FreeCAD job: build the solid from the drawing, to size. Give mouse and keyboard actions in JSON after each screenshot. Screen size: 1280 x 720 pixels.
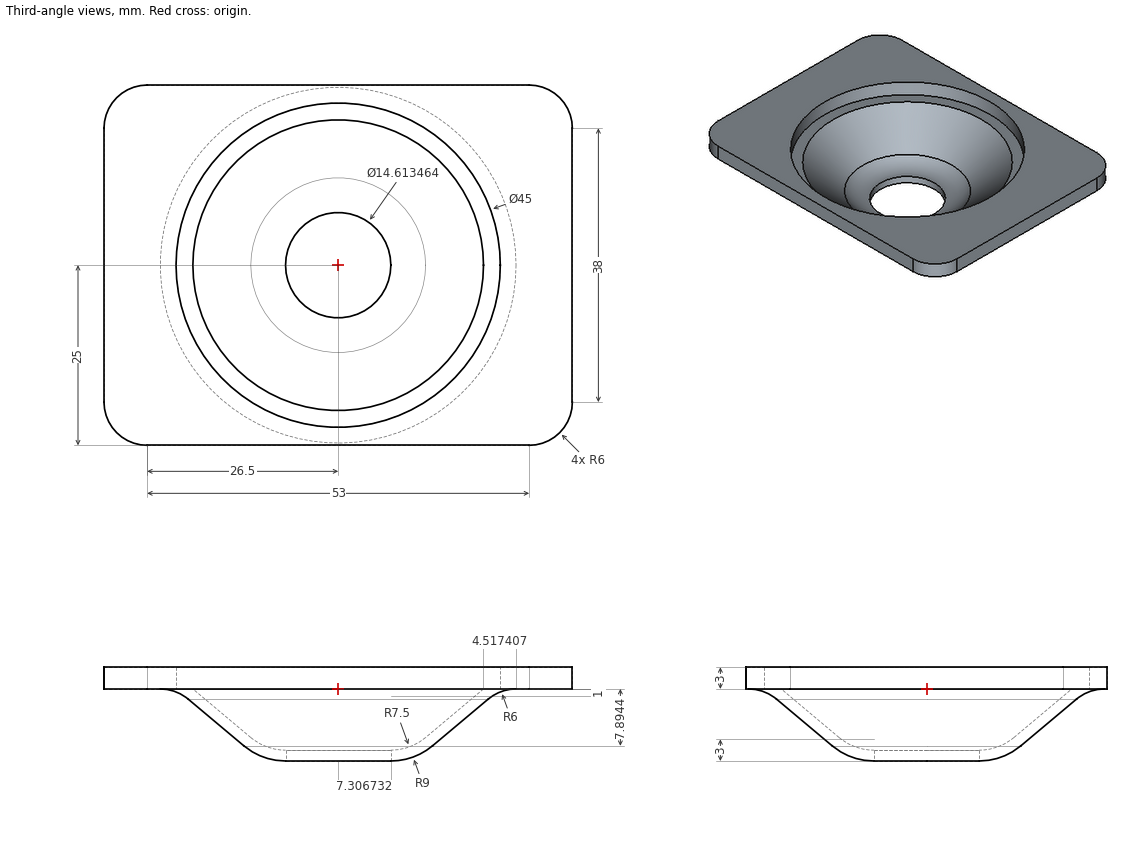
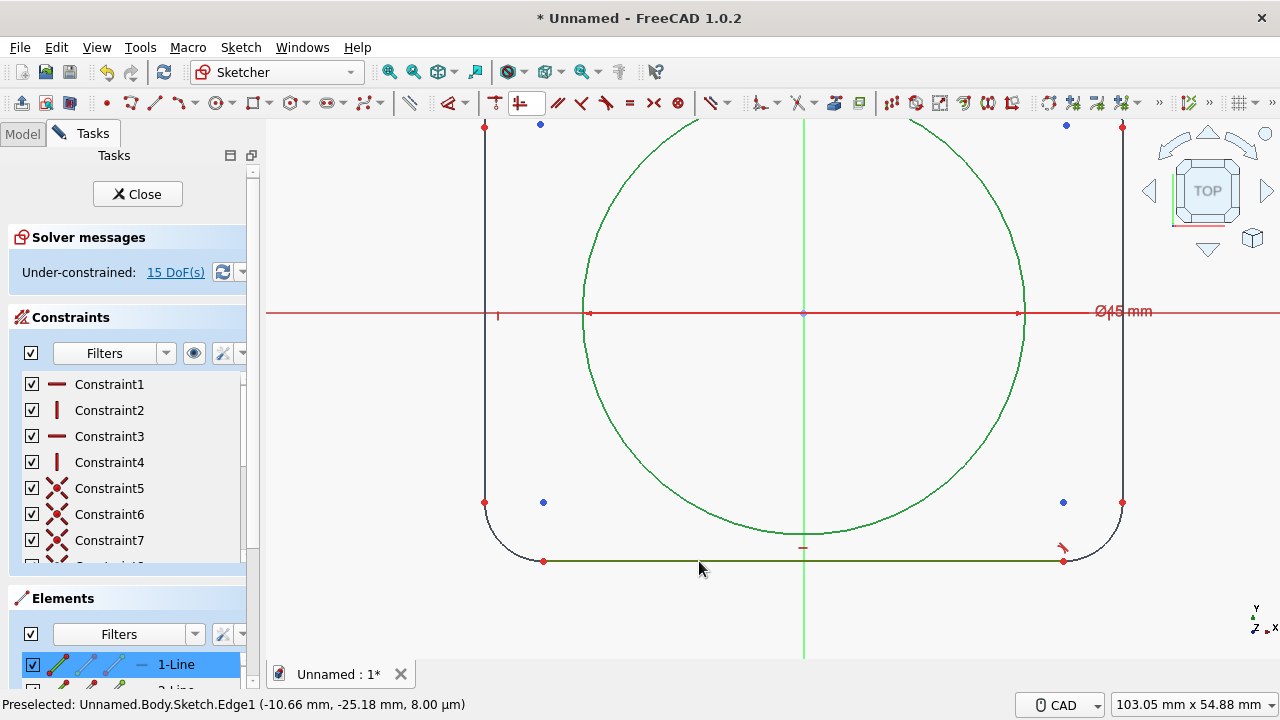
{"action": "left_click", "coordinate": [491, 529]}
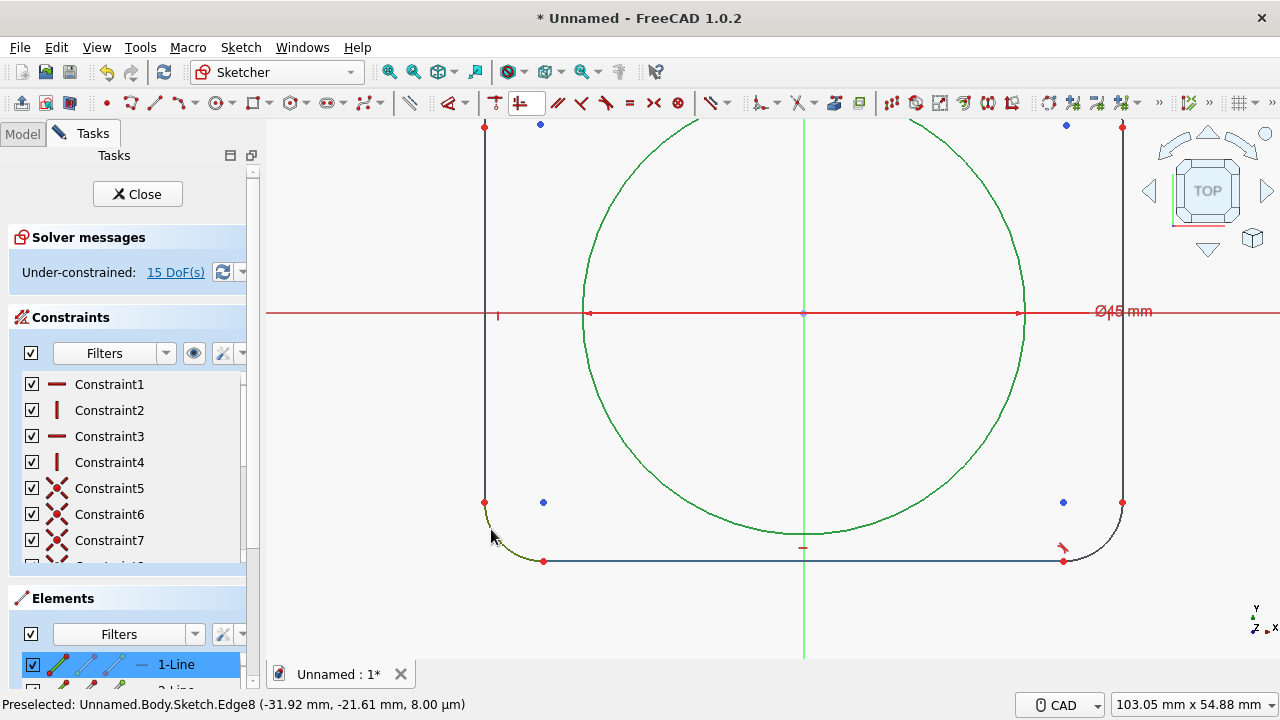
{"action": "key", "text": "t"}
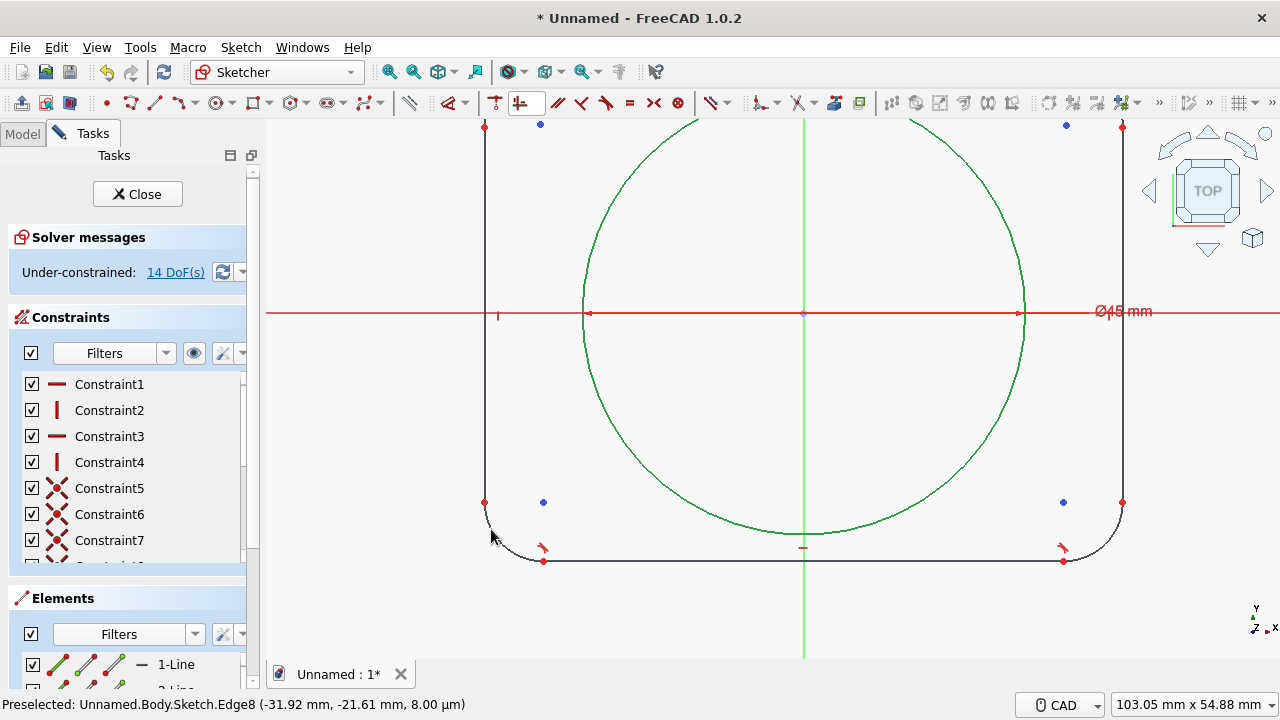
{"action": "scroll", "coordinate": [502, 543], "scroll_direction": "down", "scroll_amount": 2}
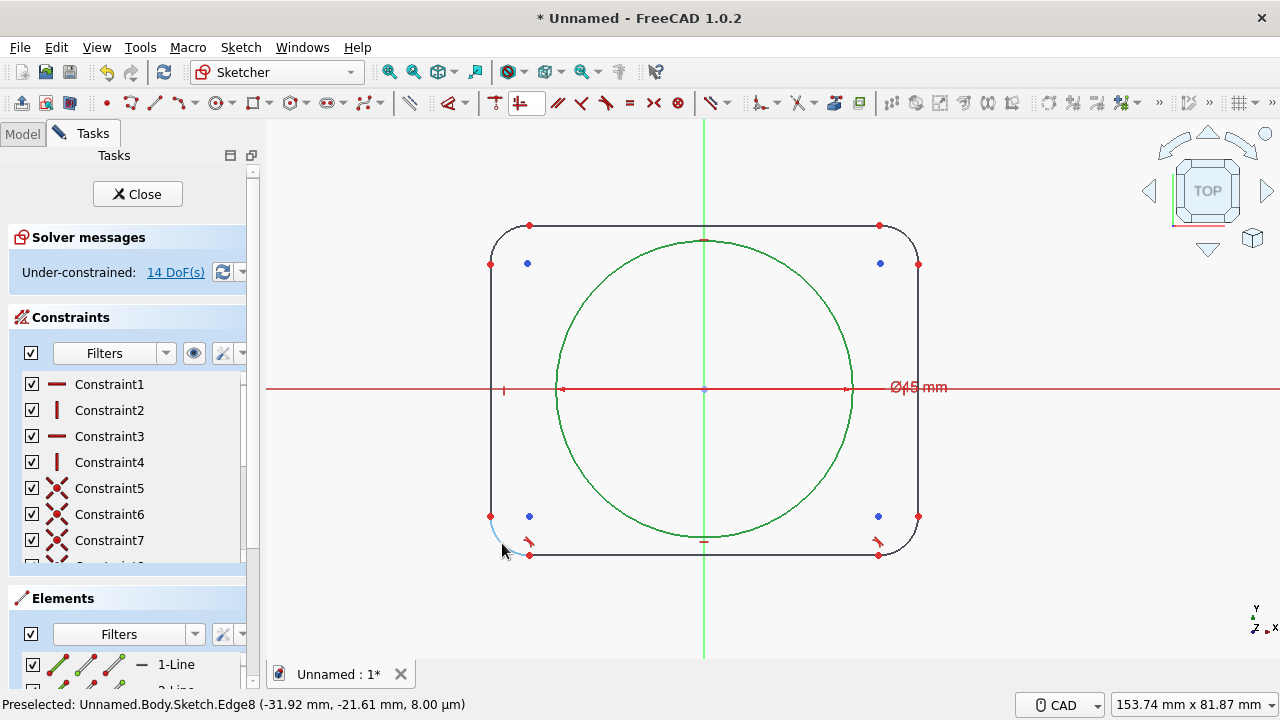
{"action": "left_click", "coordinate": [918, 441]}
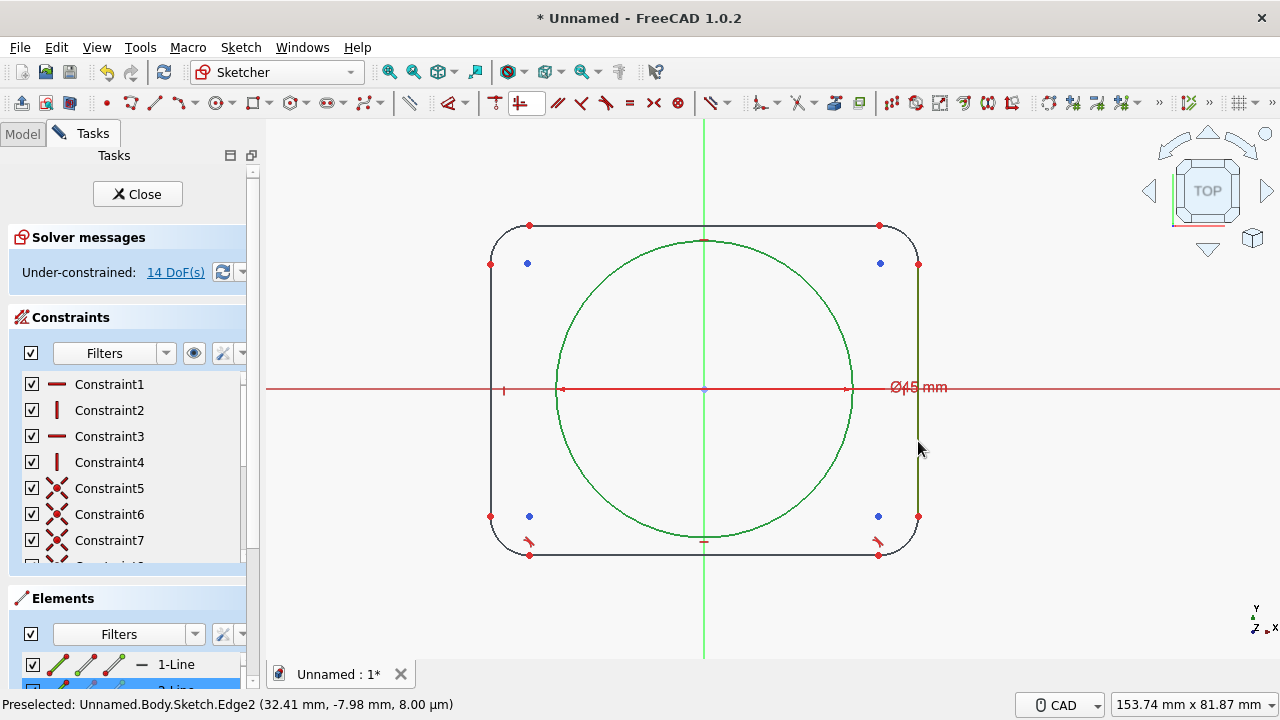
{"action": "left_click", "coordinate": [897, 551]}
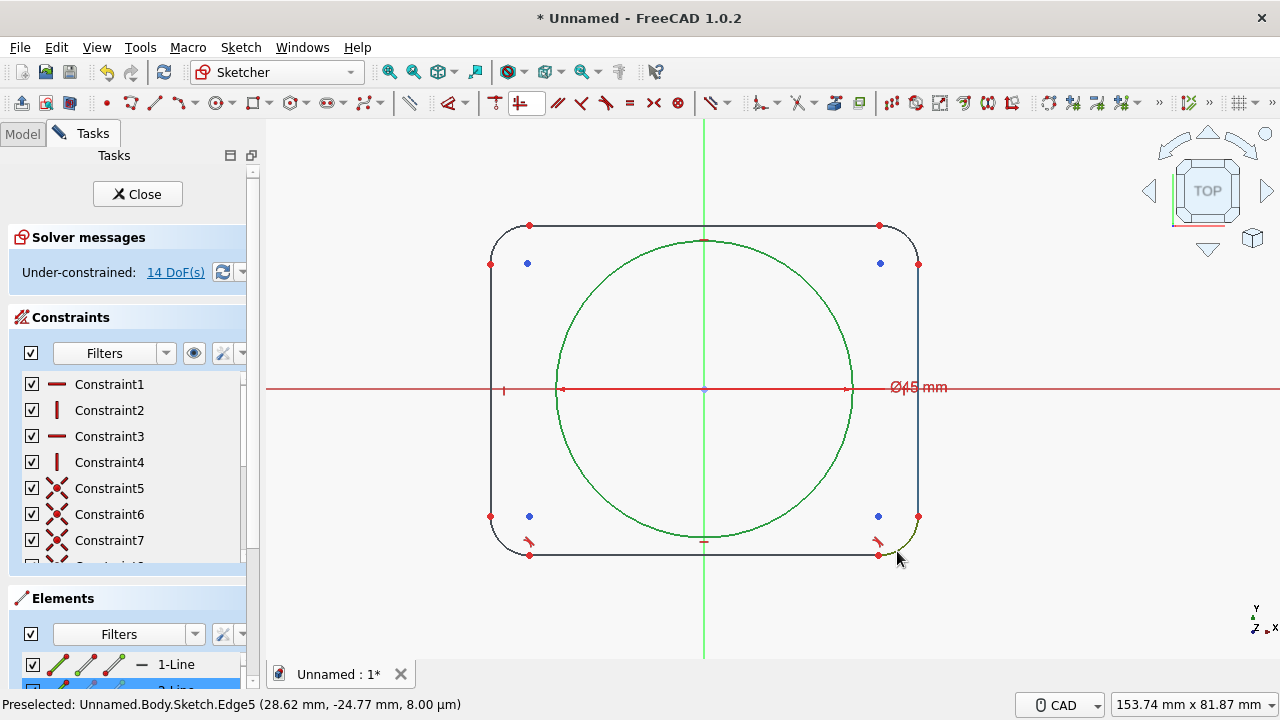
{"action": "key", "text": "t"}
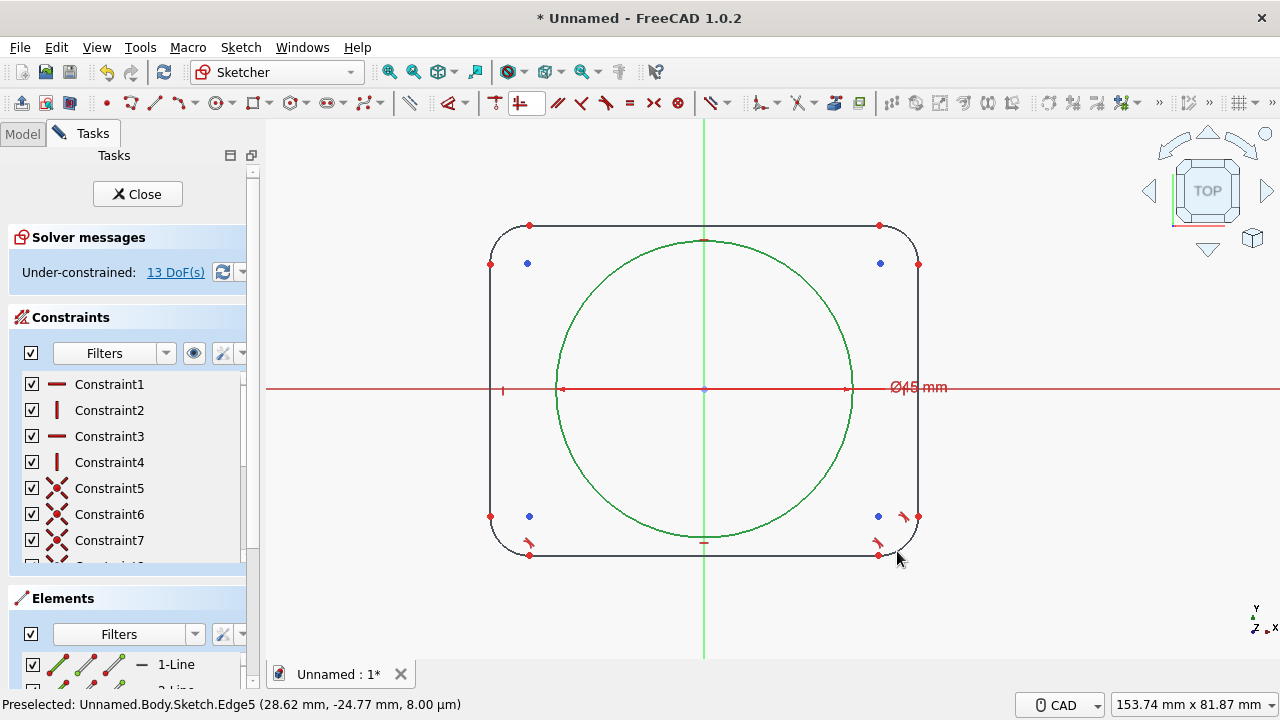
{"action": "left_click", "coordinate": [918, 441]}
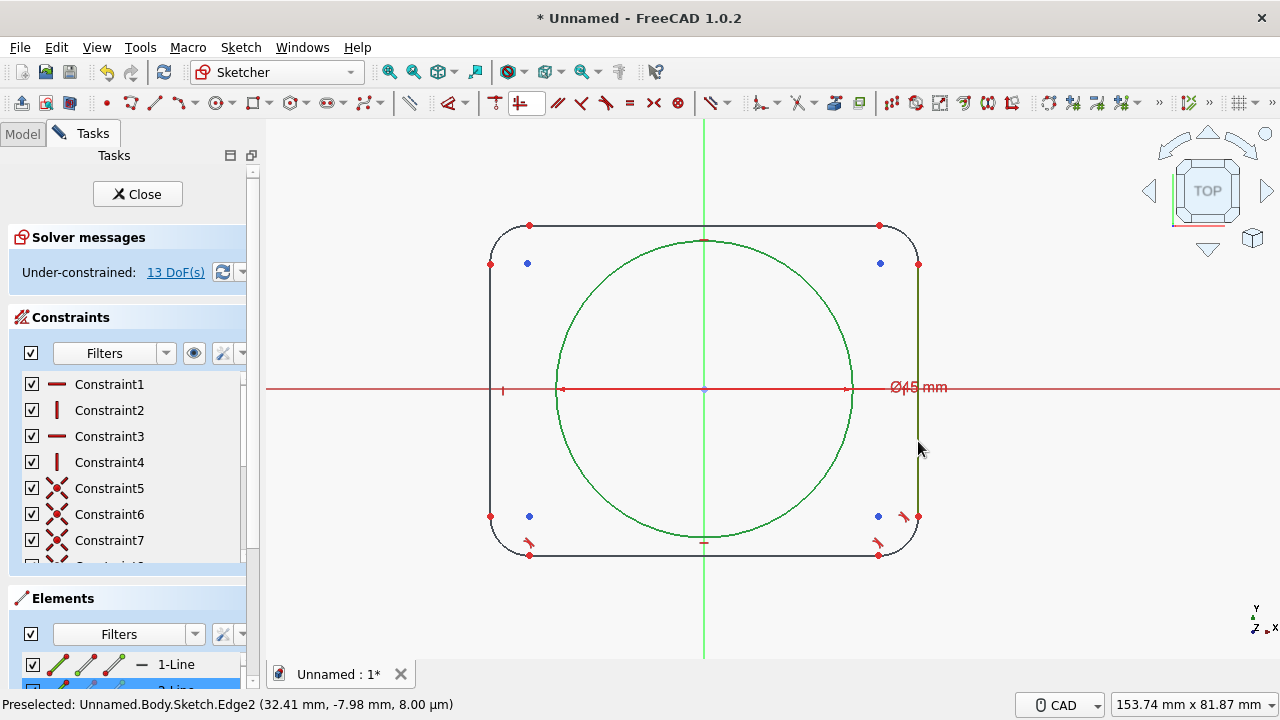
{"action": "left_click", "coordinate": [914, 247]}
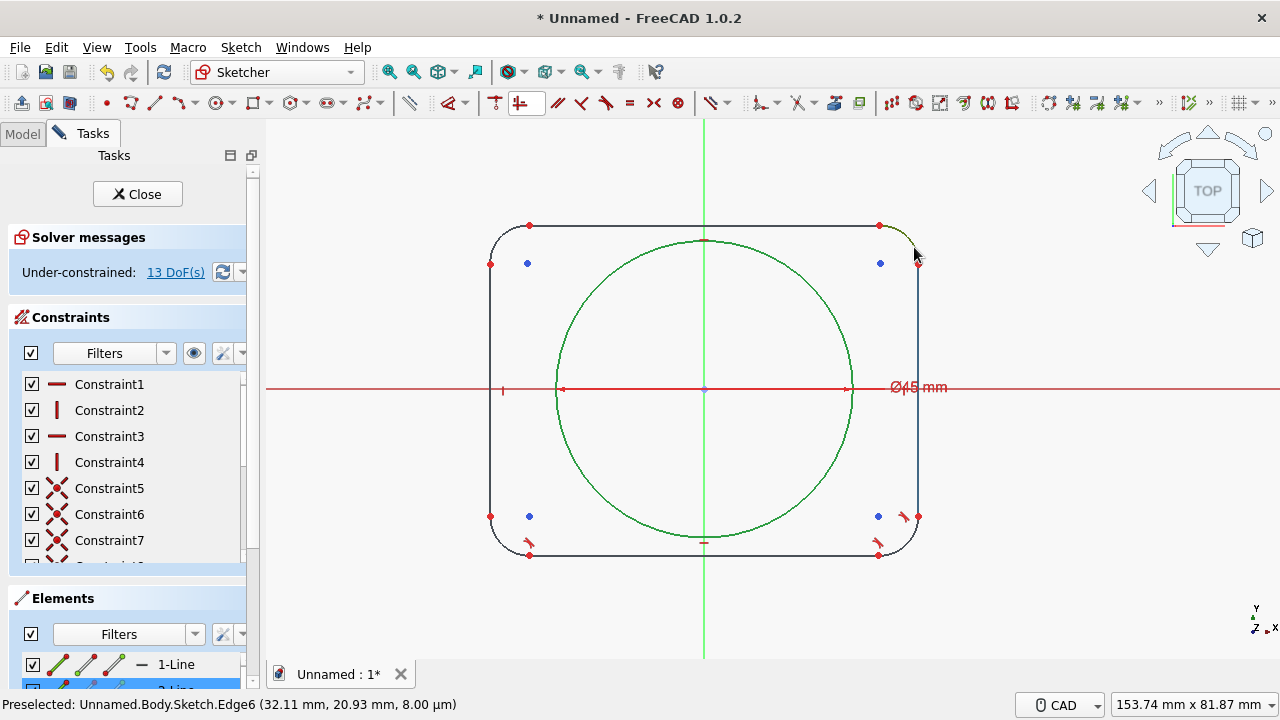
{"action": "left_click", "coordinate": [606, 104]}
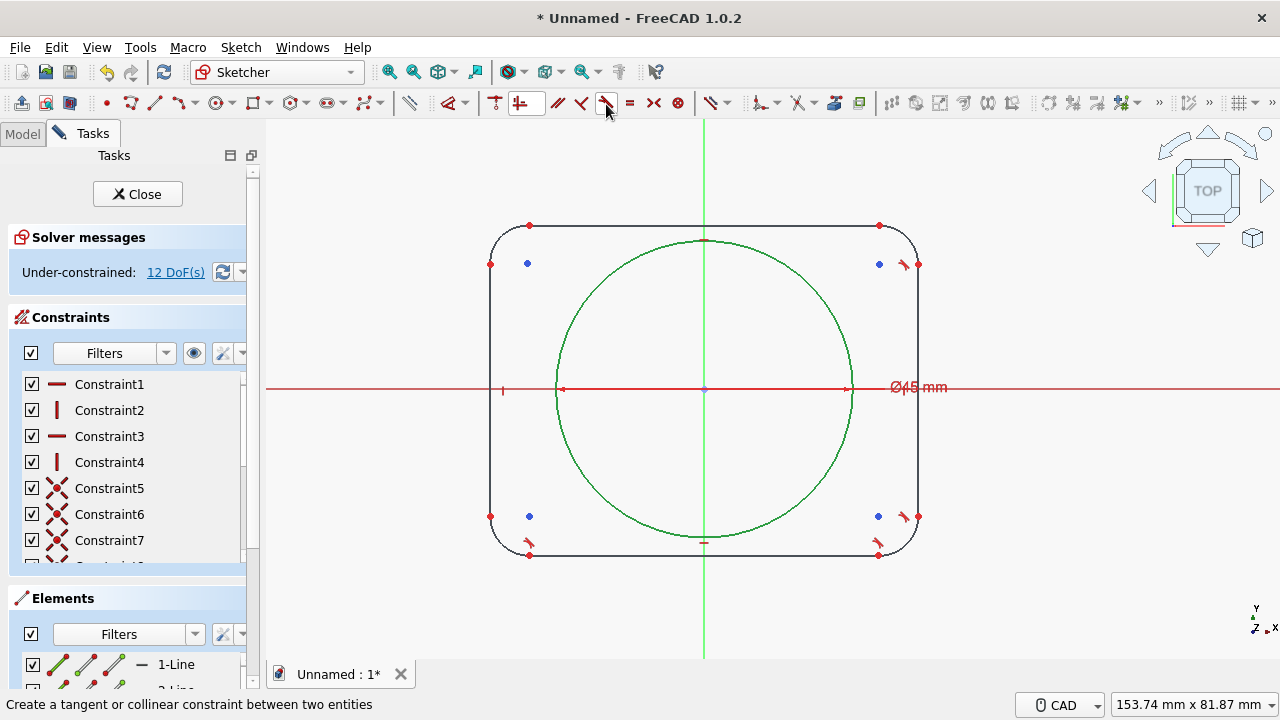
{"action": "left_click", "coordinate": [774, 226]}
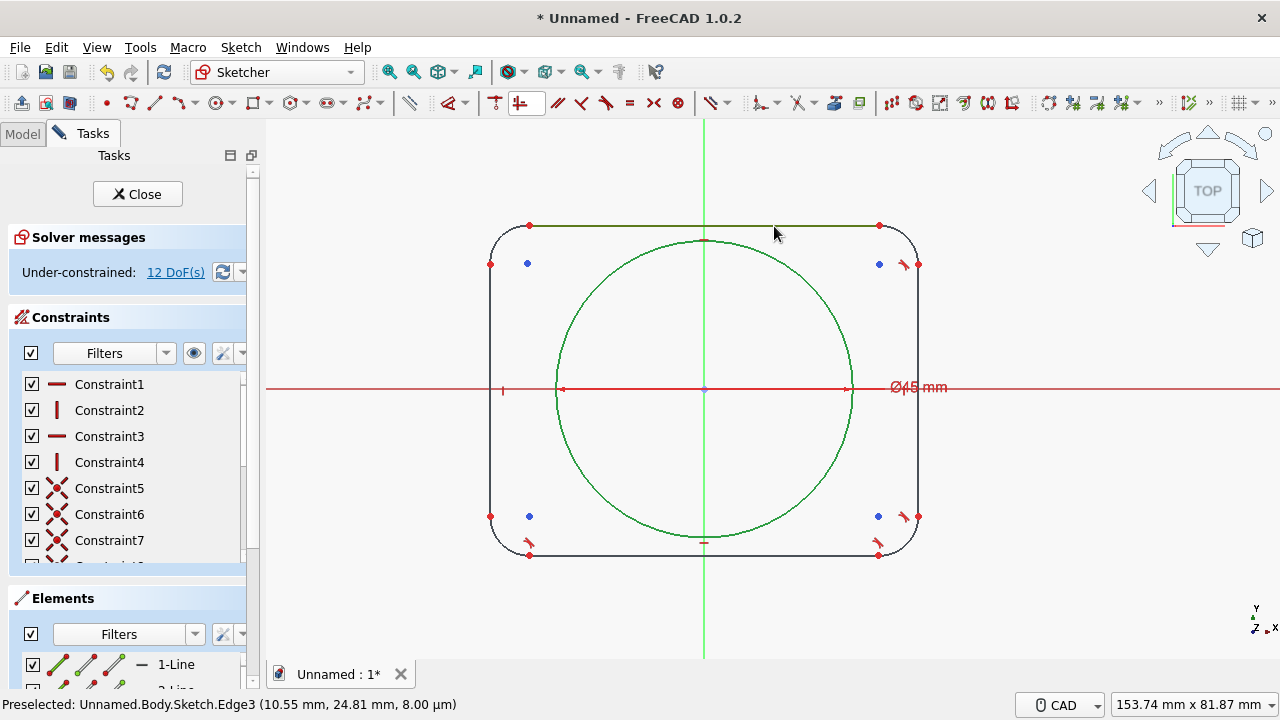
{"action": "left_click", "coordinate": [914, 247]}